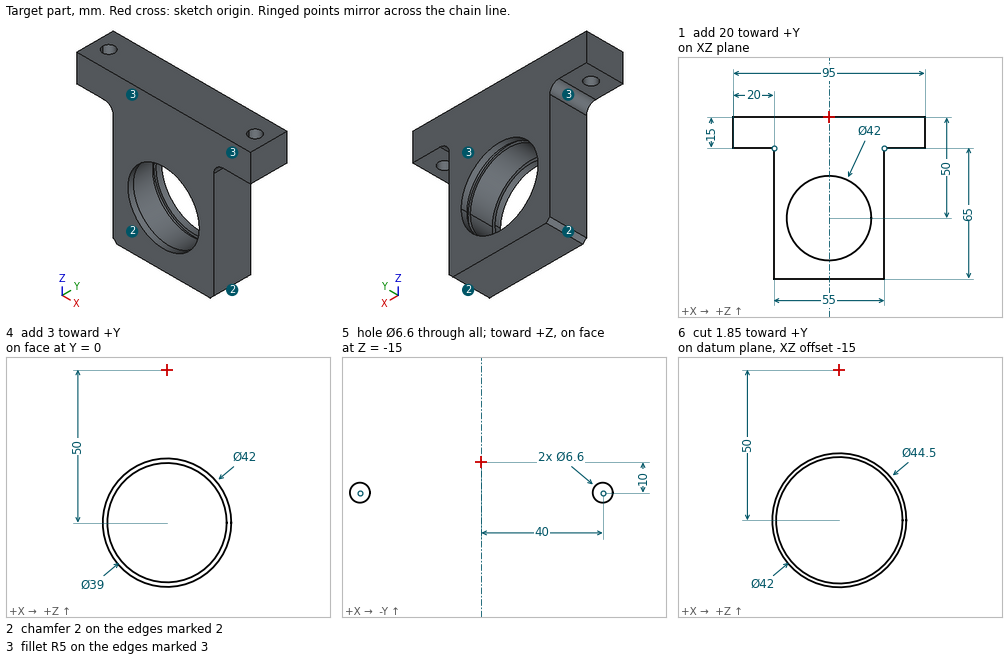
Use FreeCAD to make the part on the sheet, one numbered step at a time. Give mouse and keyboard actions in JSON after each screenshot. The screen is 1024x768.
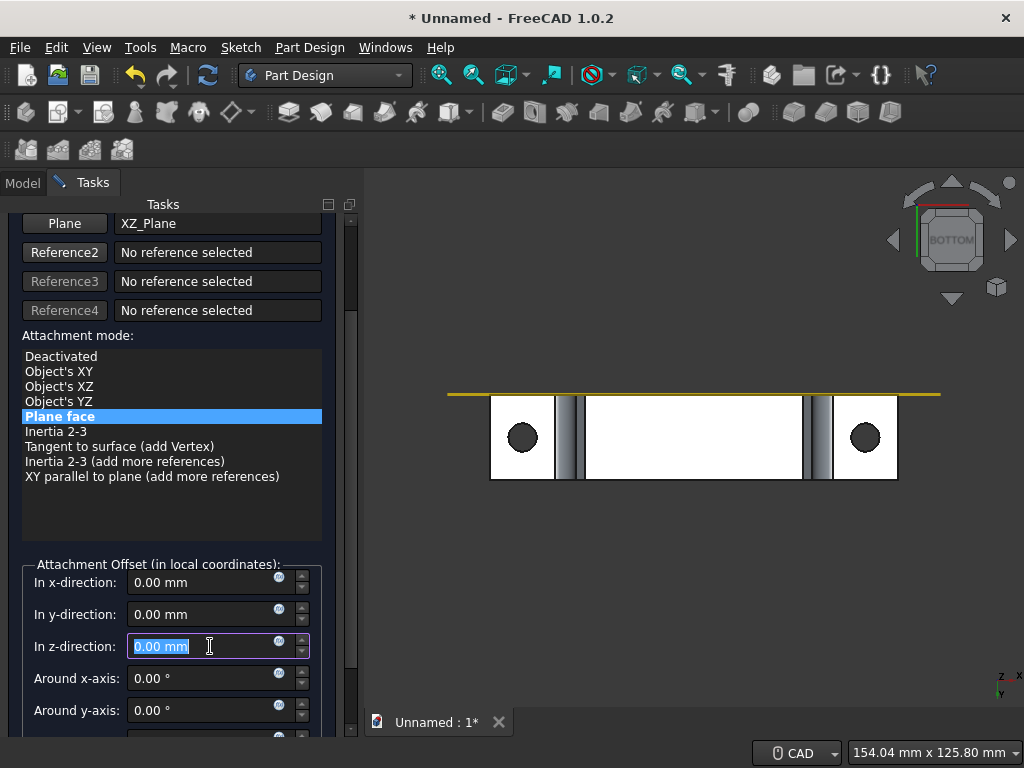
{"action": "type", "text": "-15"}
{"action": "key", "text": "Tab"}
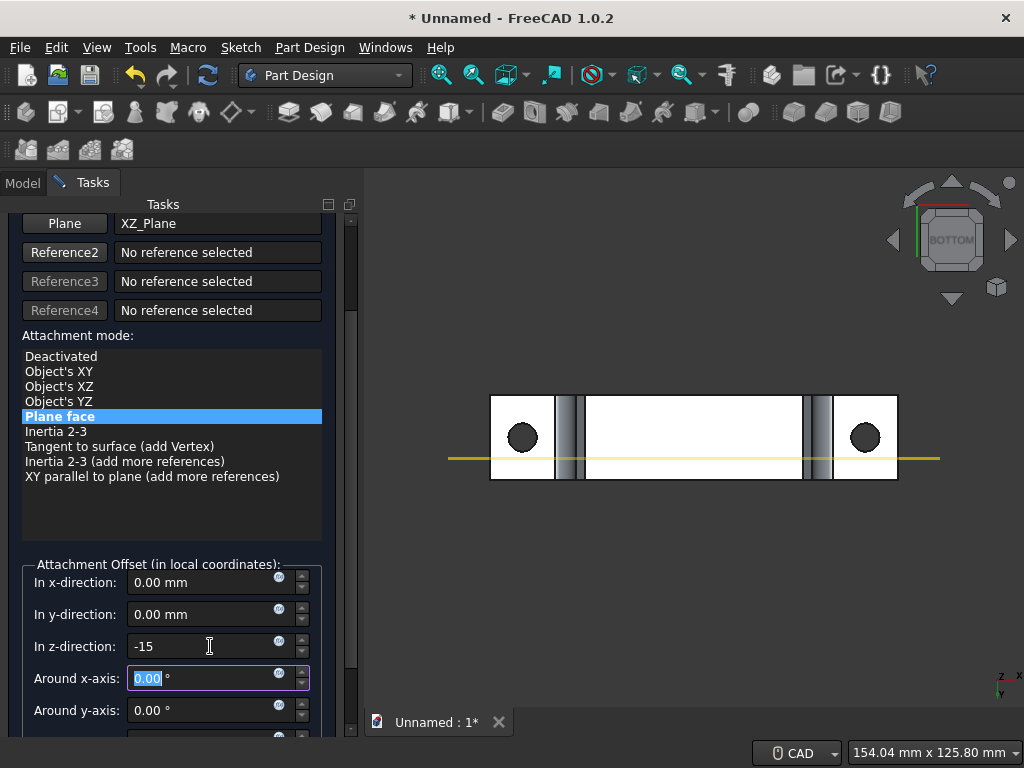
{"action": "scroll", "coordinate": [351, 475], "scroll_direction": "up", "scroll_amount": 3}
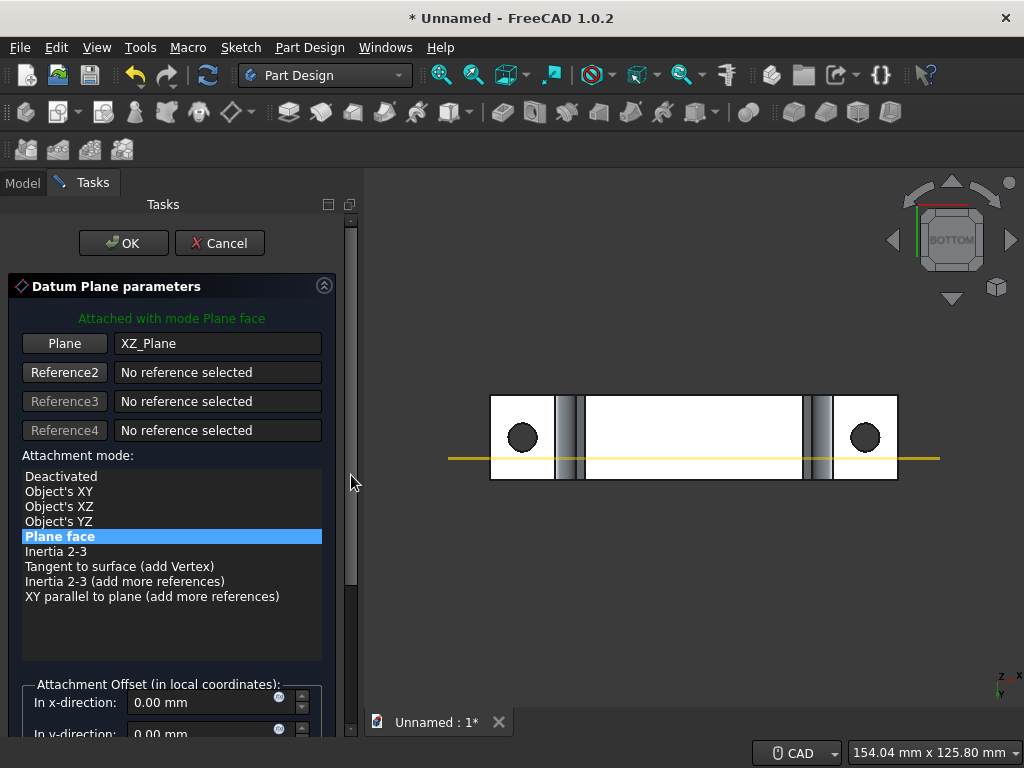
{"action": "left_click", "coordinate": [124, 243]}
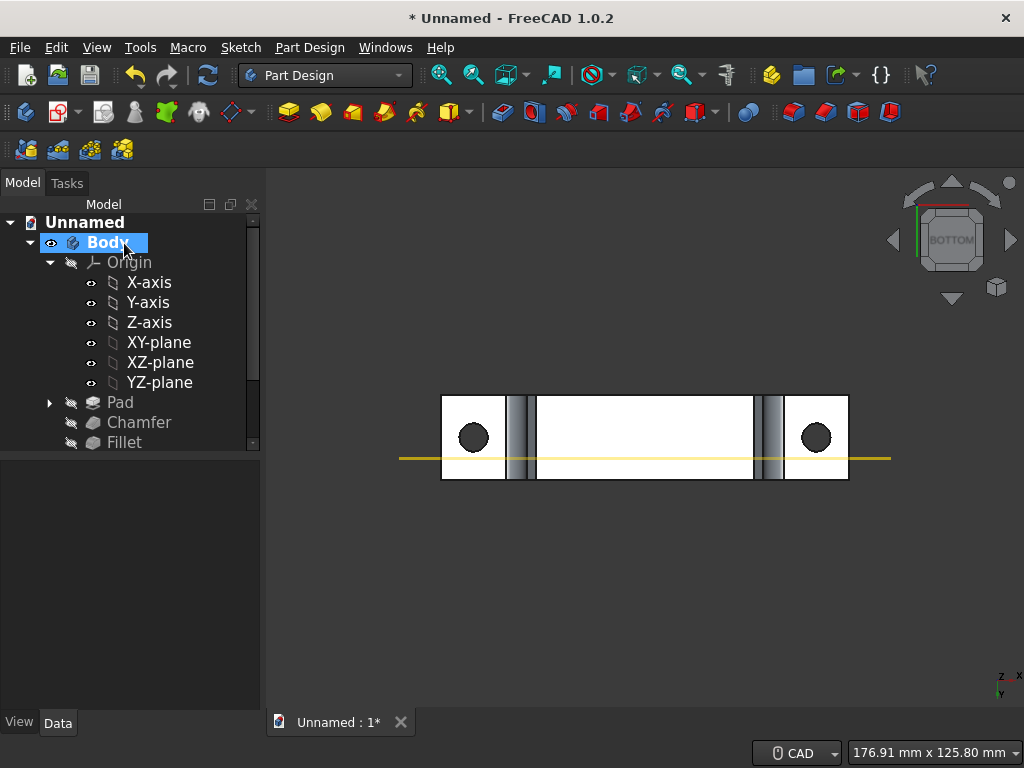
{"action": "scroll", "coordinate": [100, 338], "scroll_direction": "down", "scroll_amount": 3}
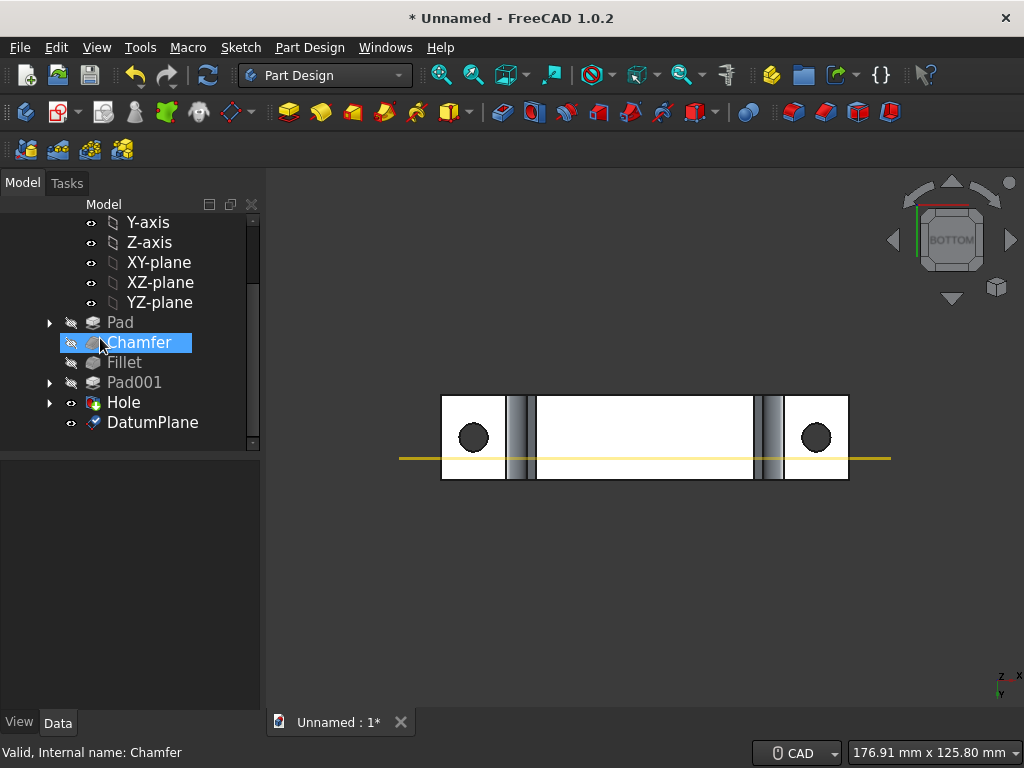
{"action": "left_click", "coordinate": [116, 423]}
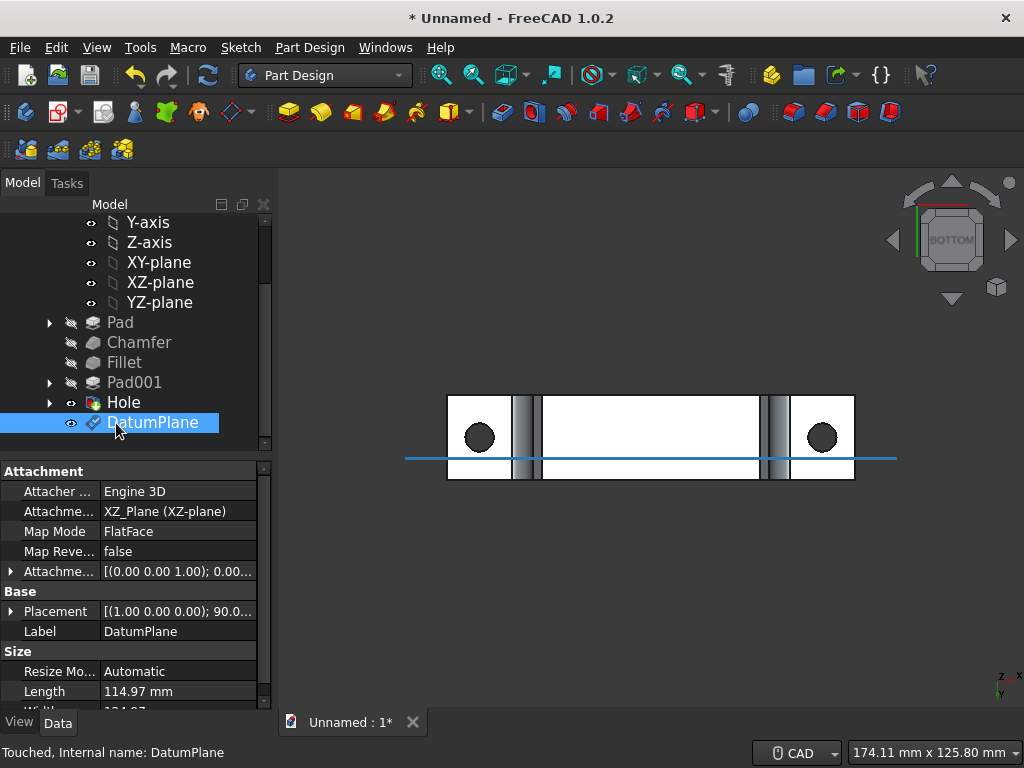
{"action": "left_click", "coordinate": [58, 112]}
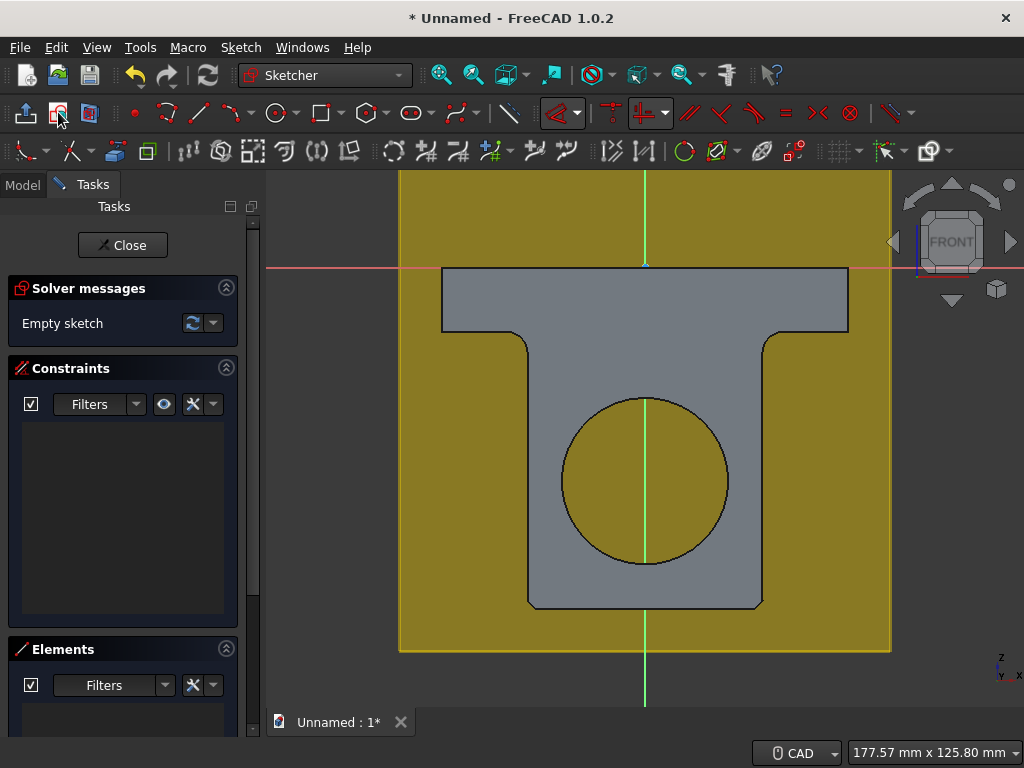
{"action": "left_click", "coordinate": [90, 114]}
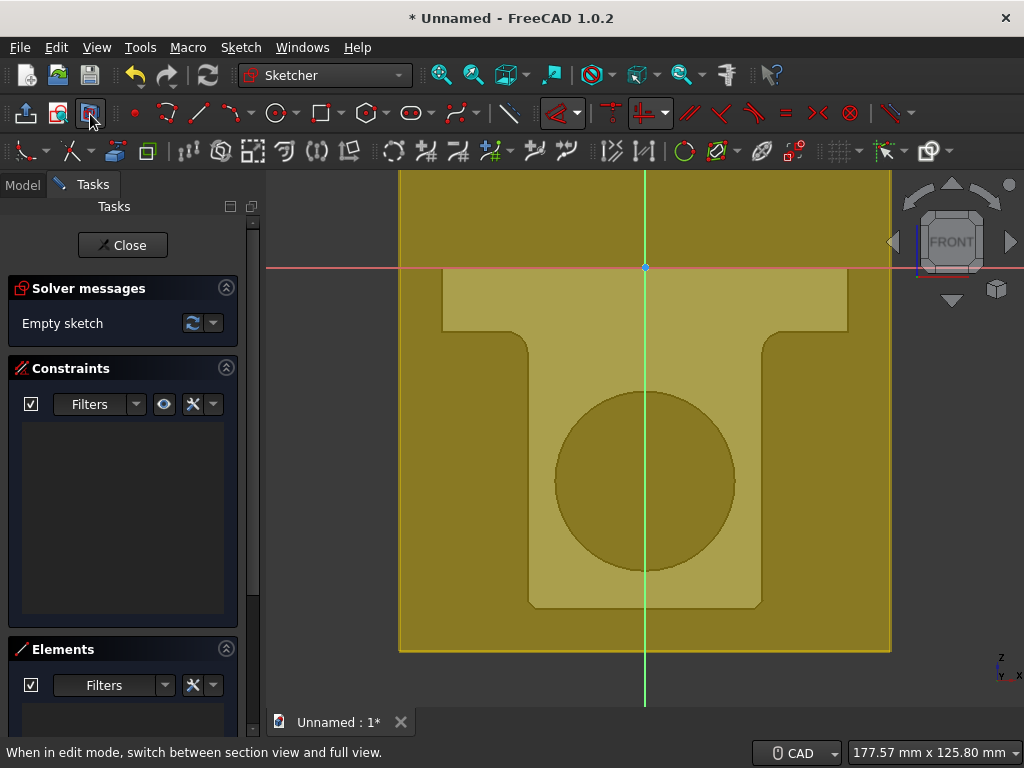
{"action": "left_click", "coordinate": [276, 114]}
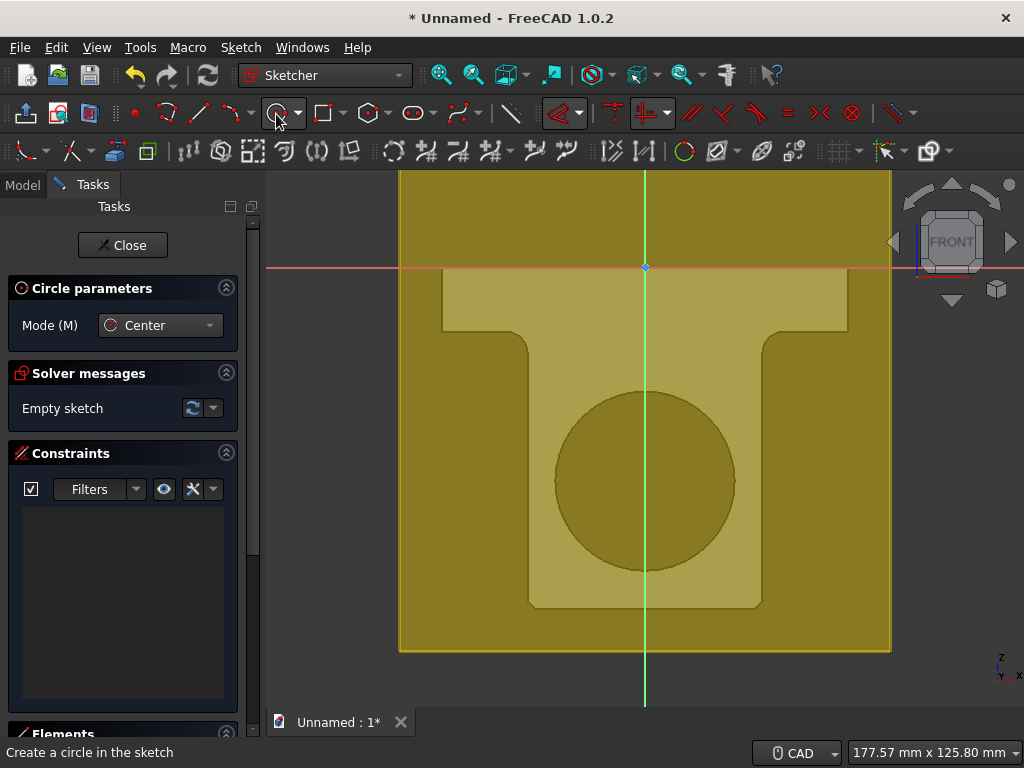
{"action": "left_click", "coordinate": [645, 481]}
{"action": "mouse_move", "coordinate": [712, 414]}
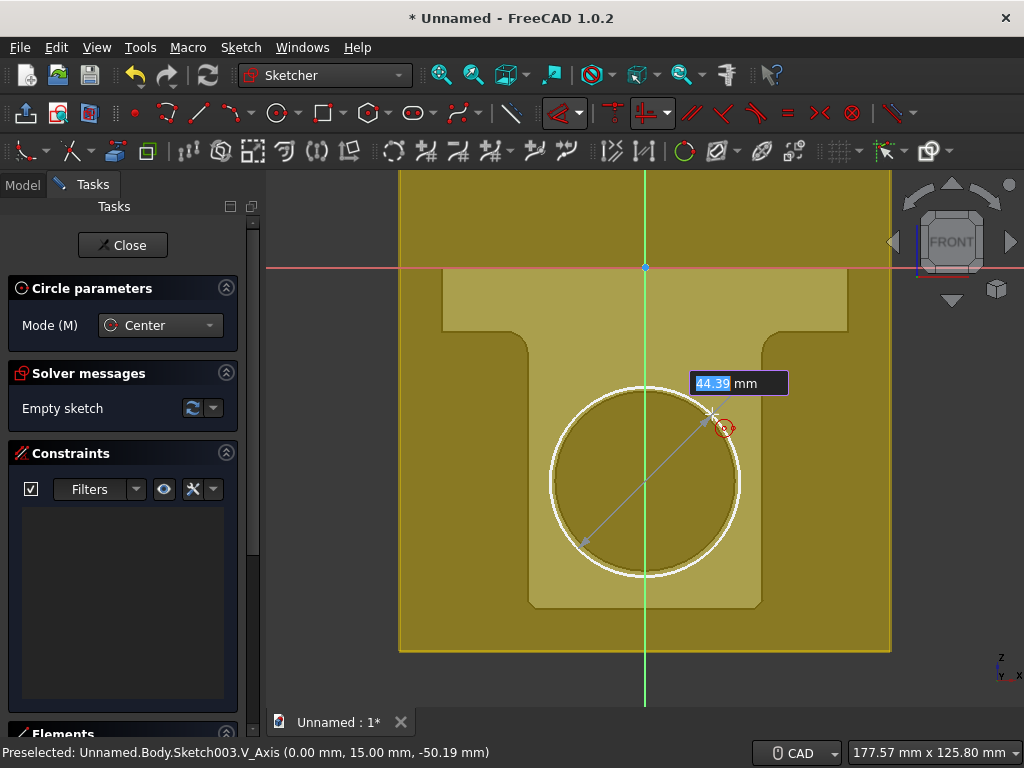
{"action": "type", "text": "44.5"}
{"action": "key", "text": "Return"}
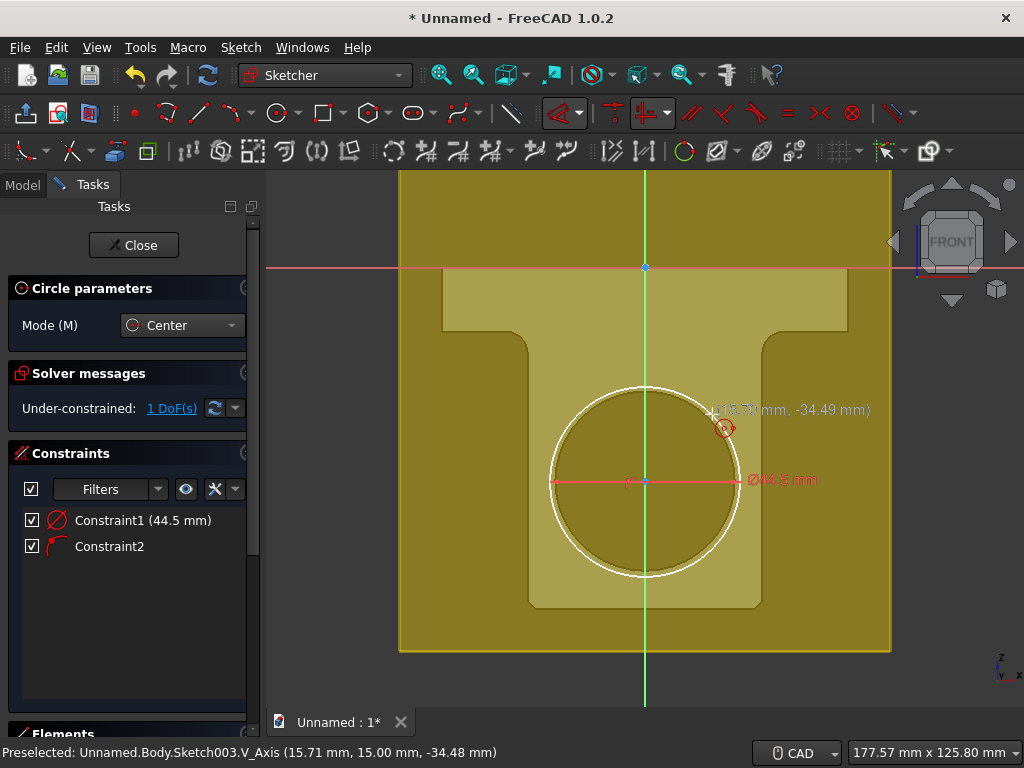
{"action": "left_click", "coordinate": [645, 482]}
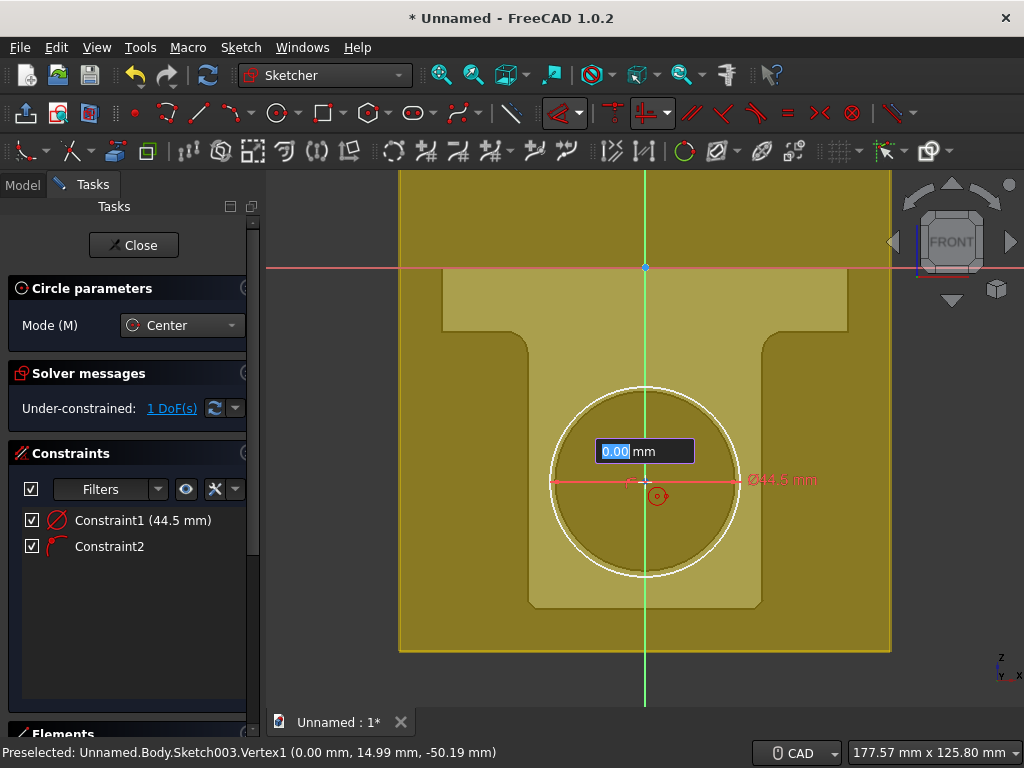
{"action": "scroll", "coordinate": [614, 565], "scroll_direction": "up", "scroll_amount": 6}
{"action": "mouse_move", "coordinate": [614, 565]}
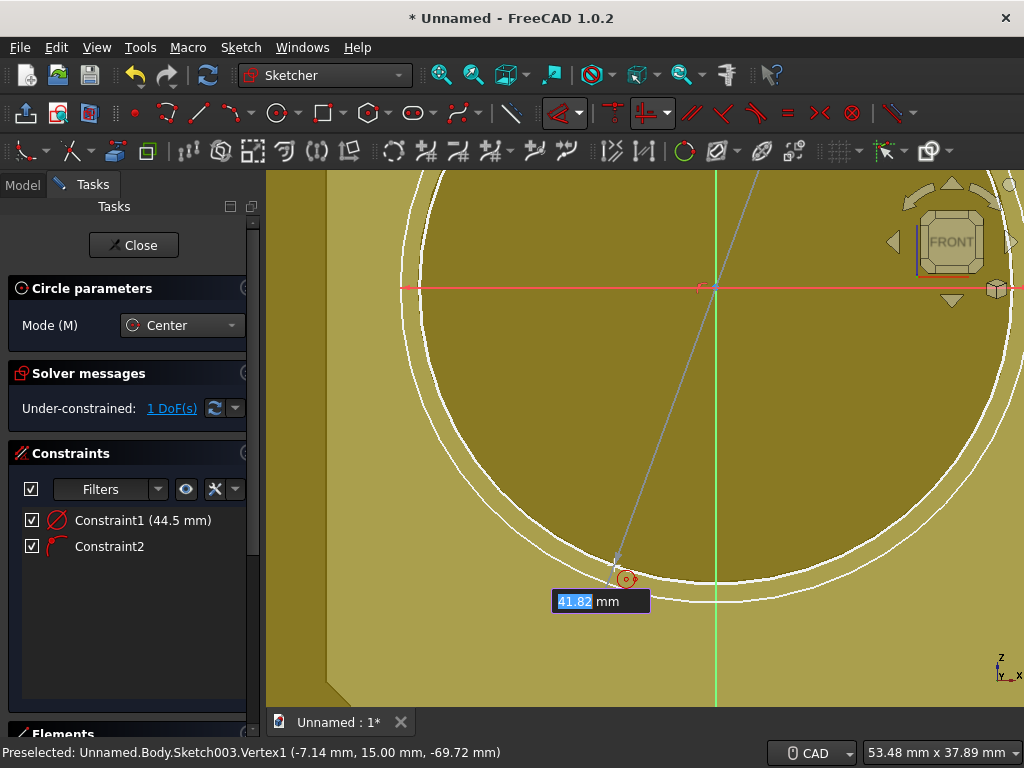
{"action": "type", "text": "42"}
{"action": "key", "text": "Return"}
{"action": "key", "text": "Escape"}